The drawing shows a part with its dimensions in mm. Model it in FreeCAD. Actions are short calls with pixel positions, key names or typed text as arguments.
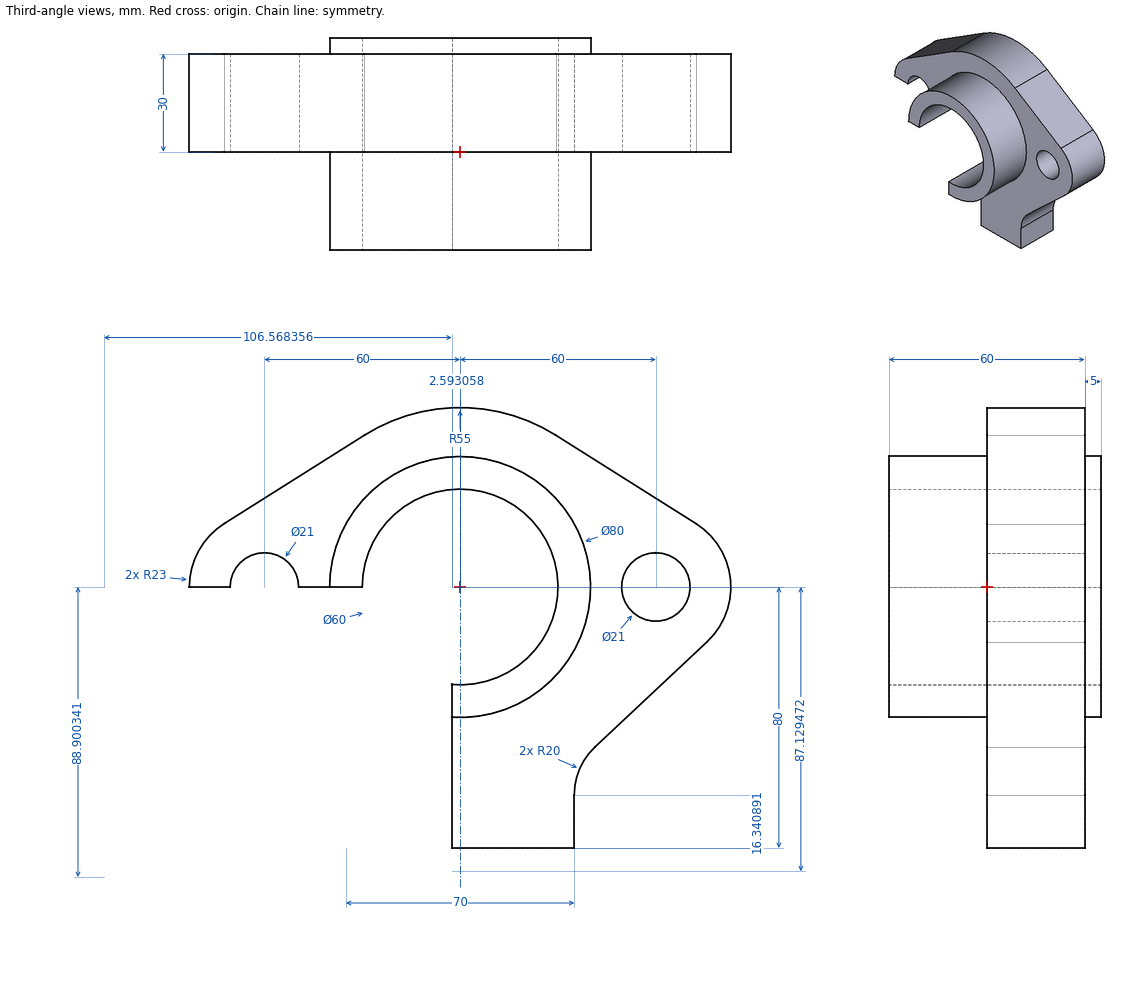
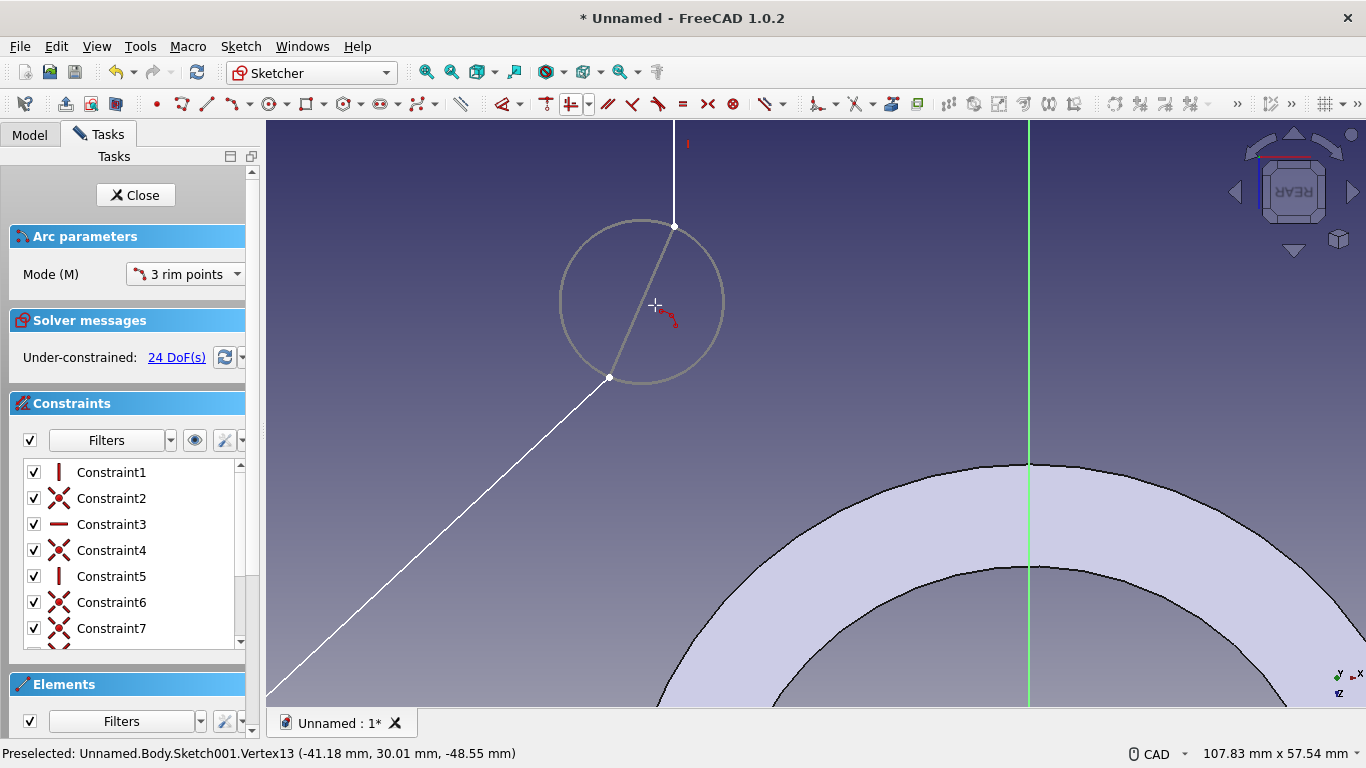
click(656, 304)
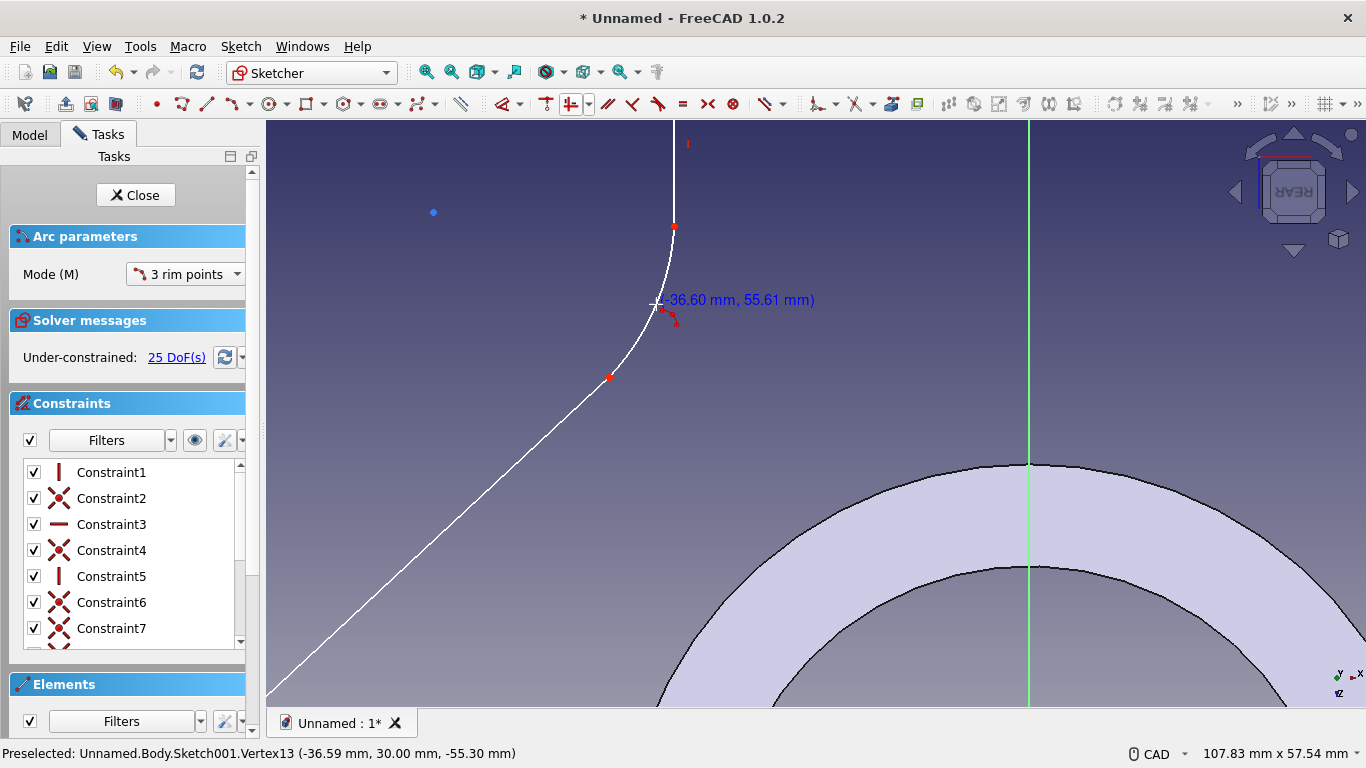
scroll(655, 305, down, 7)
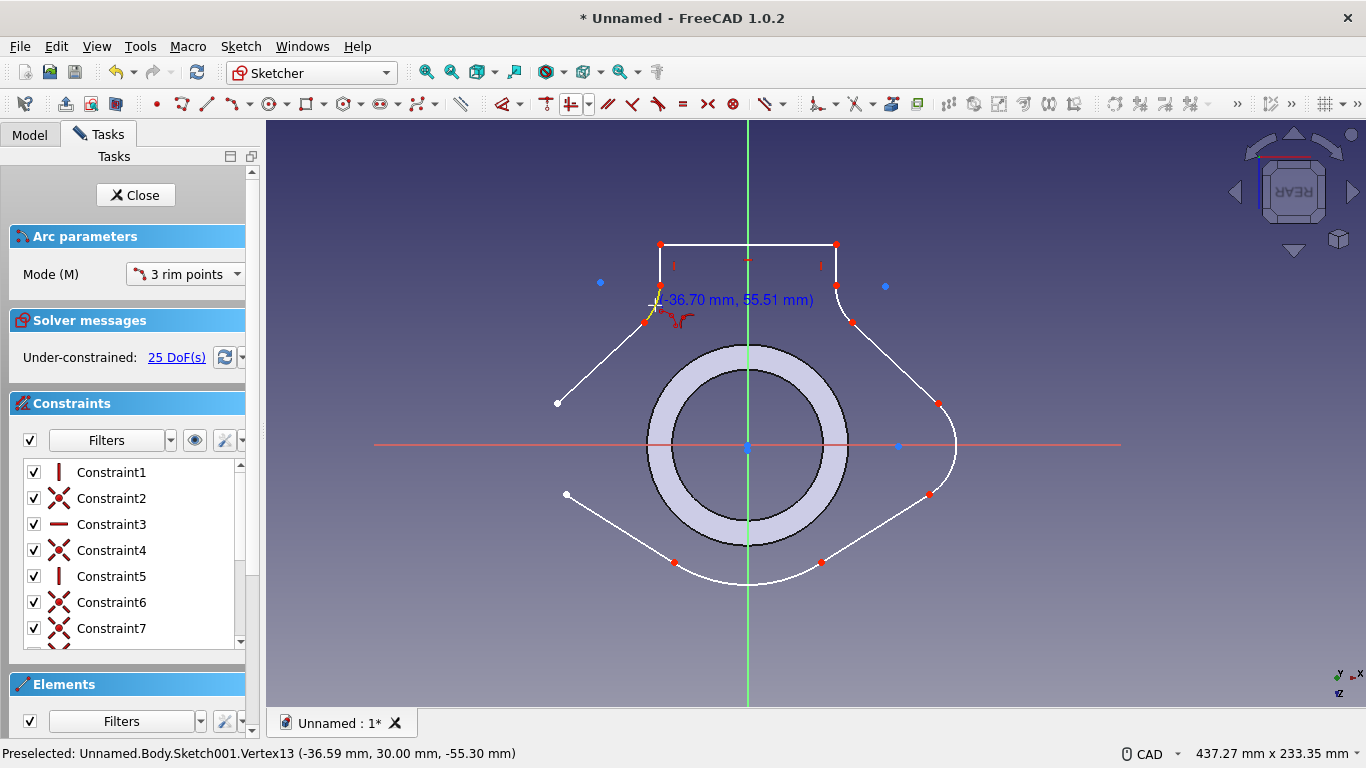
click(557, 404)
click(566, 495)
click(541, 461)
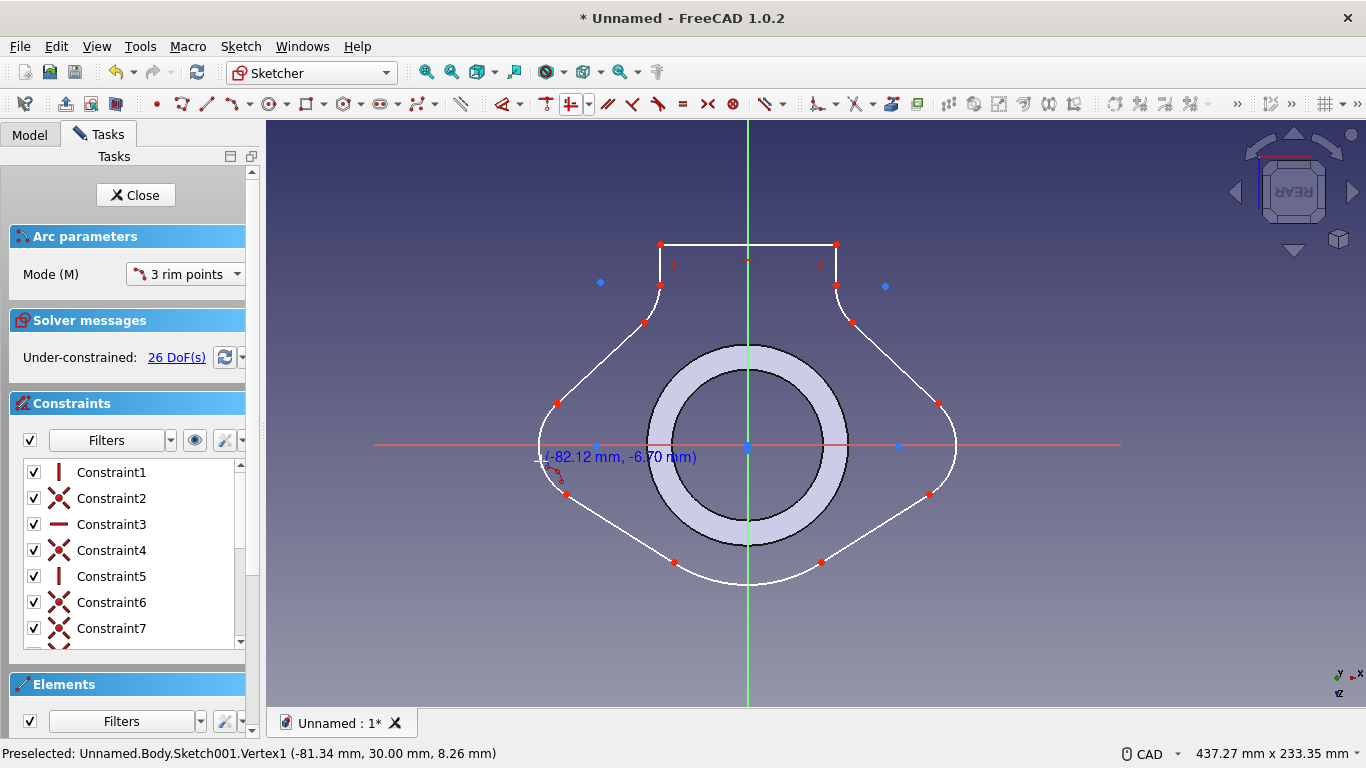
click(268, 104)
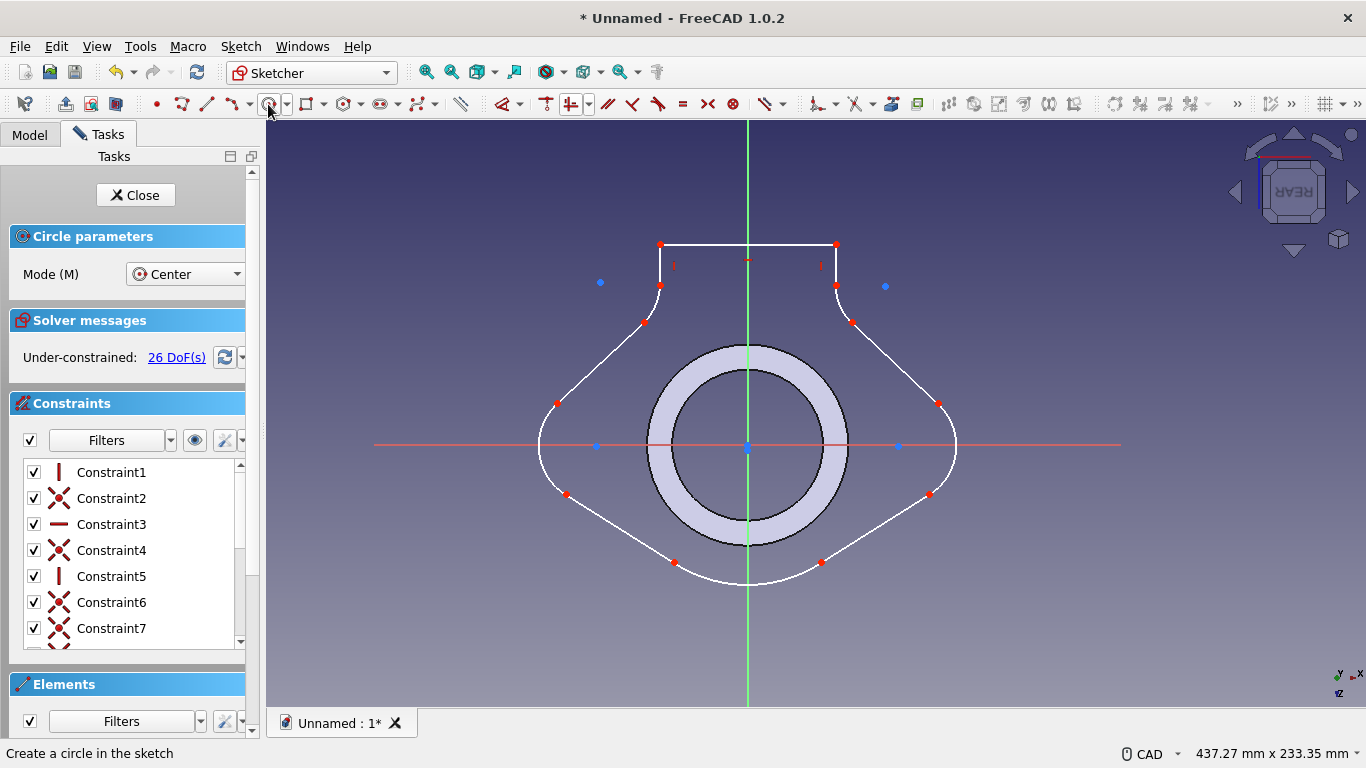
click(748, 445)
move(819, 374)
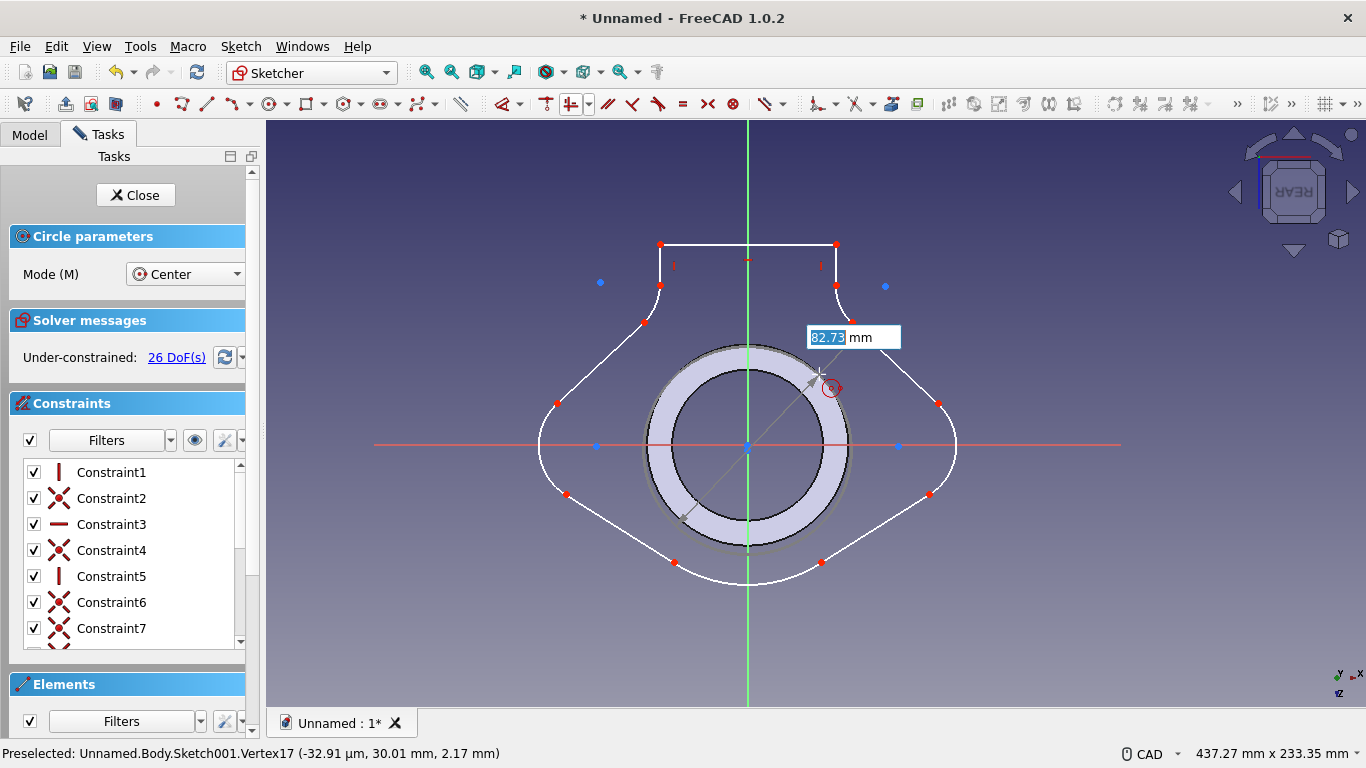
text(80)
key(Return)
key(Escape)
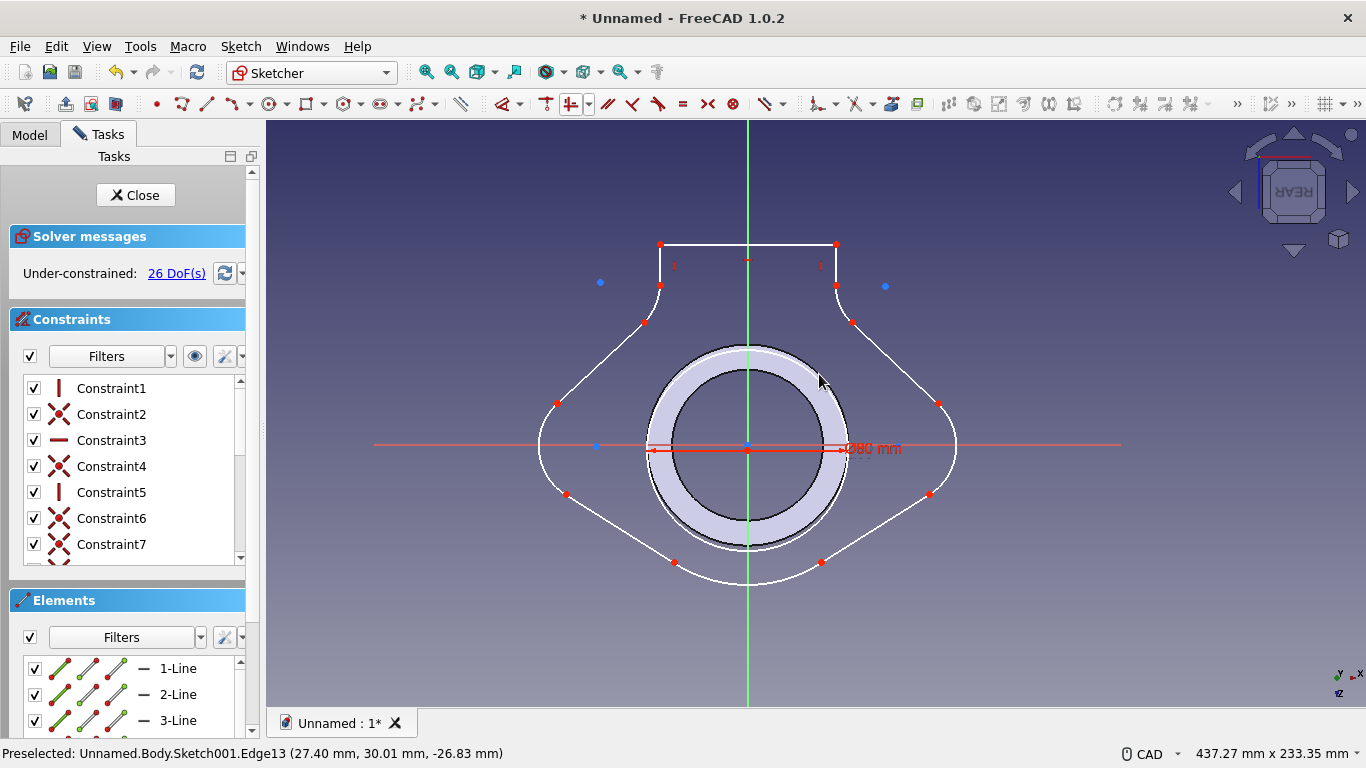
click(598, 515)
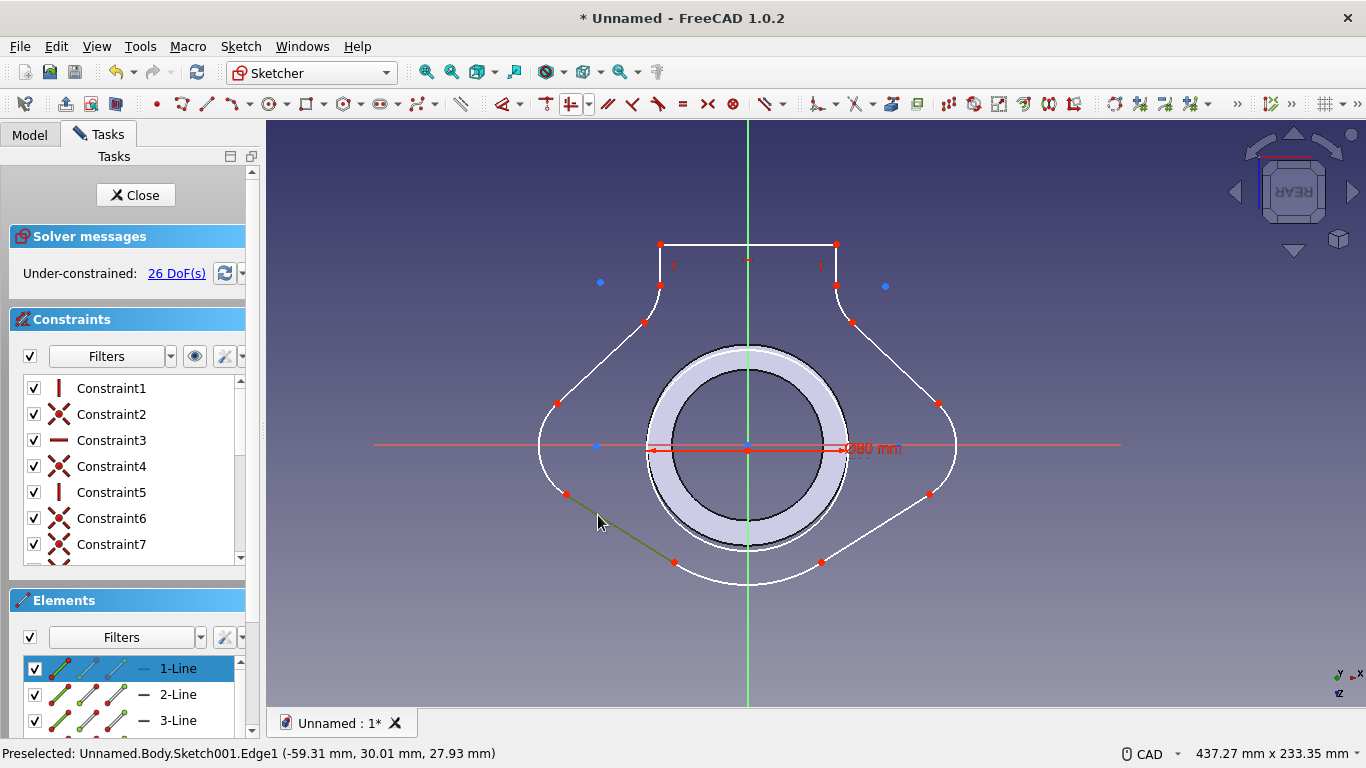
click(717, 581)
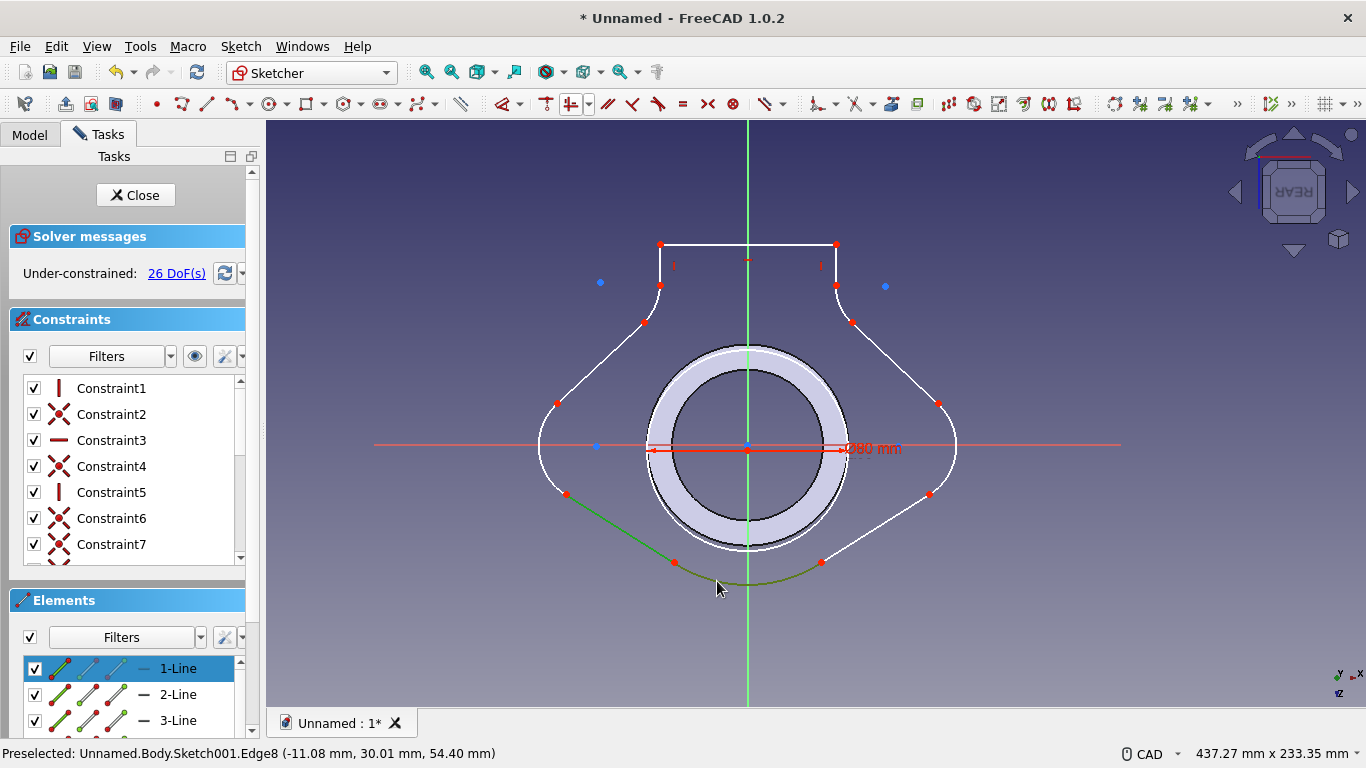
click(658, 104)